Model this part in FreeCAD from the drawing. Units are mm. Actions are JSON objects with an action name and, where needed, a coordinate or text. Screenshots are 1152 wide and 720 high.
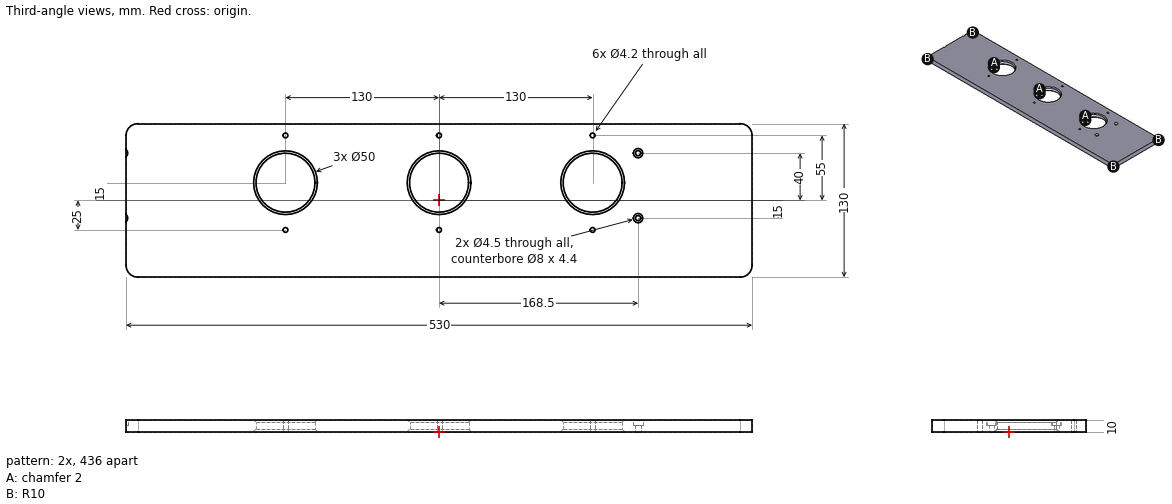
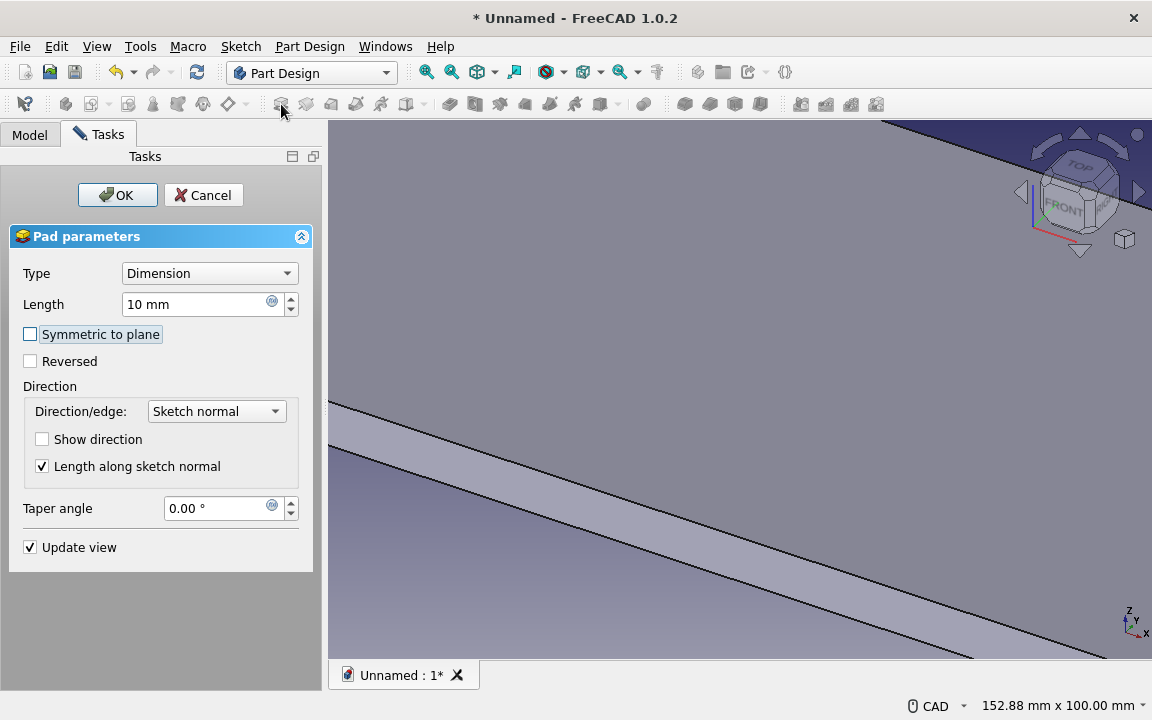
{"action": "left_click", "coordinate": [118, 195]}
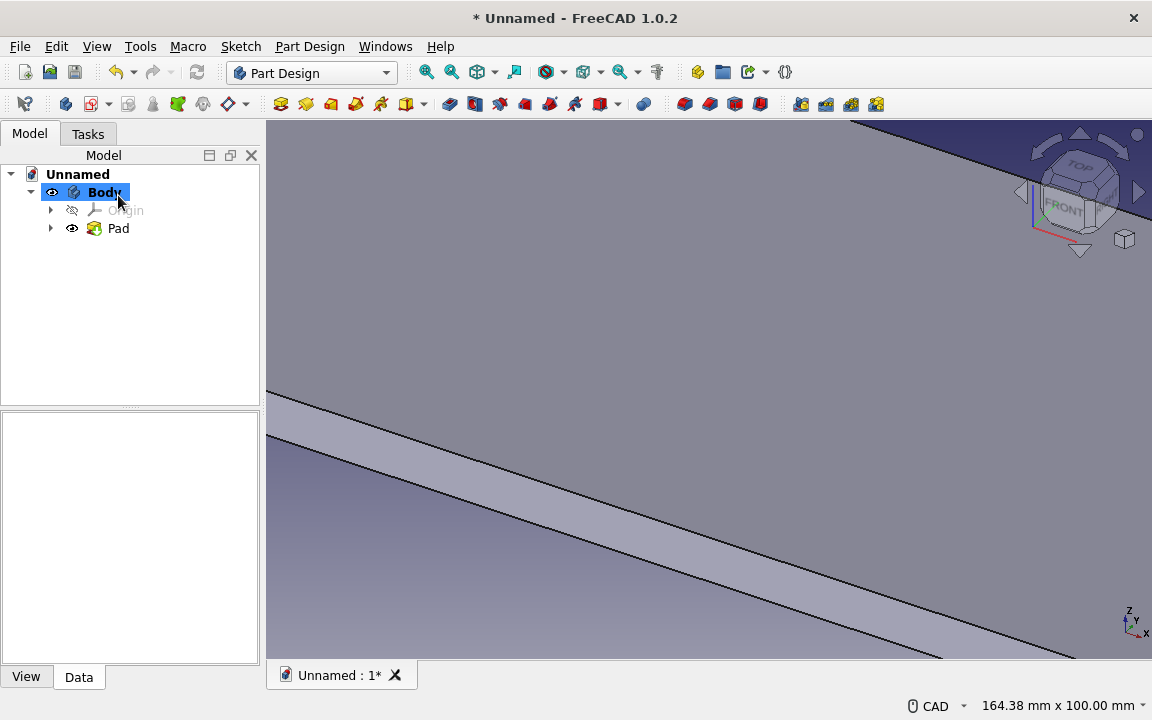
{"action": "left_click", "coordinate": [427, 72]}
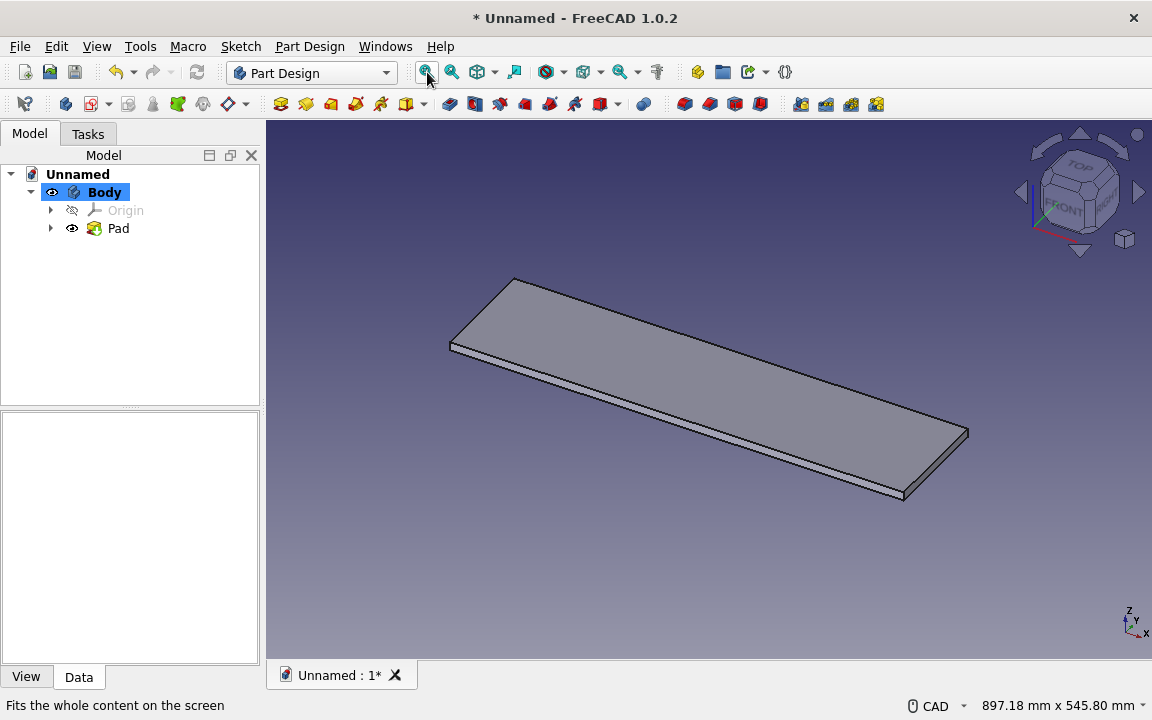
{"action": "left_click", "coordinate": [839, 427]}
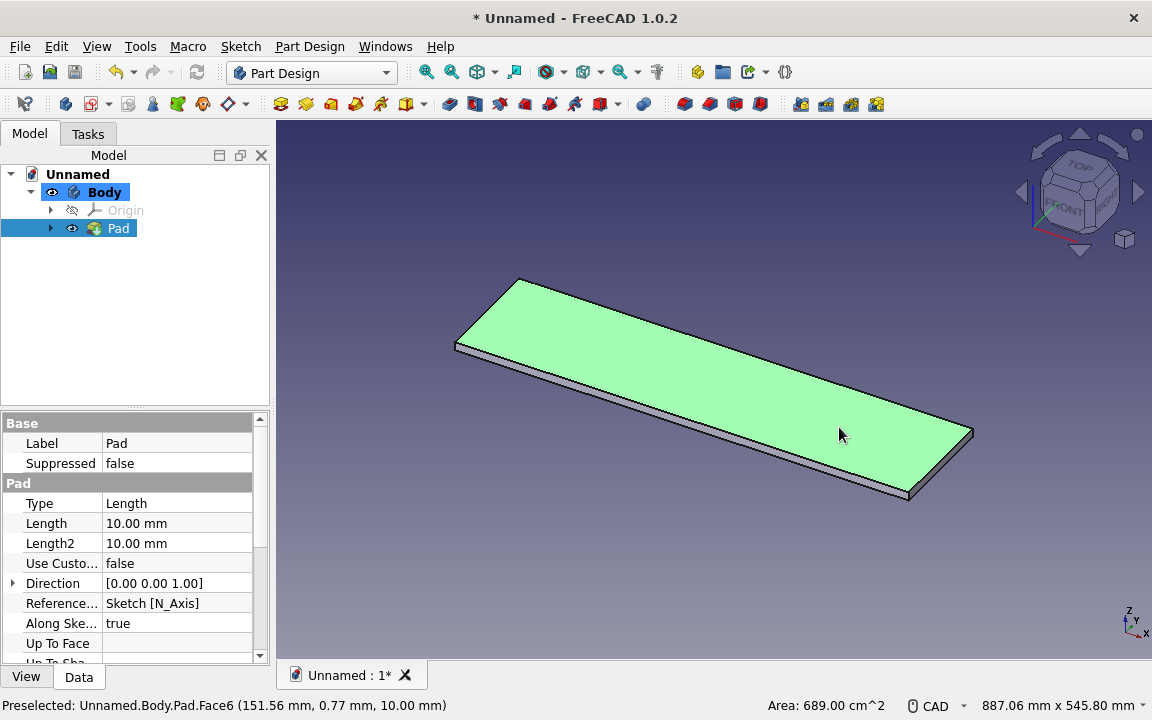
{"action": "left_click", "coordinate": [90, 104]}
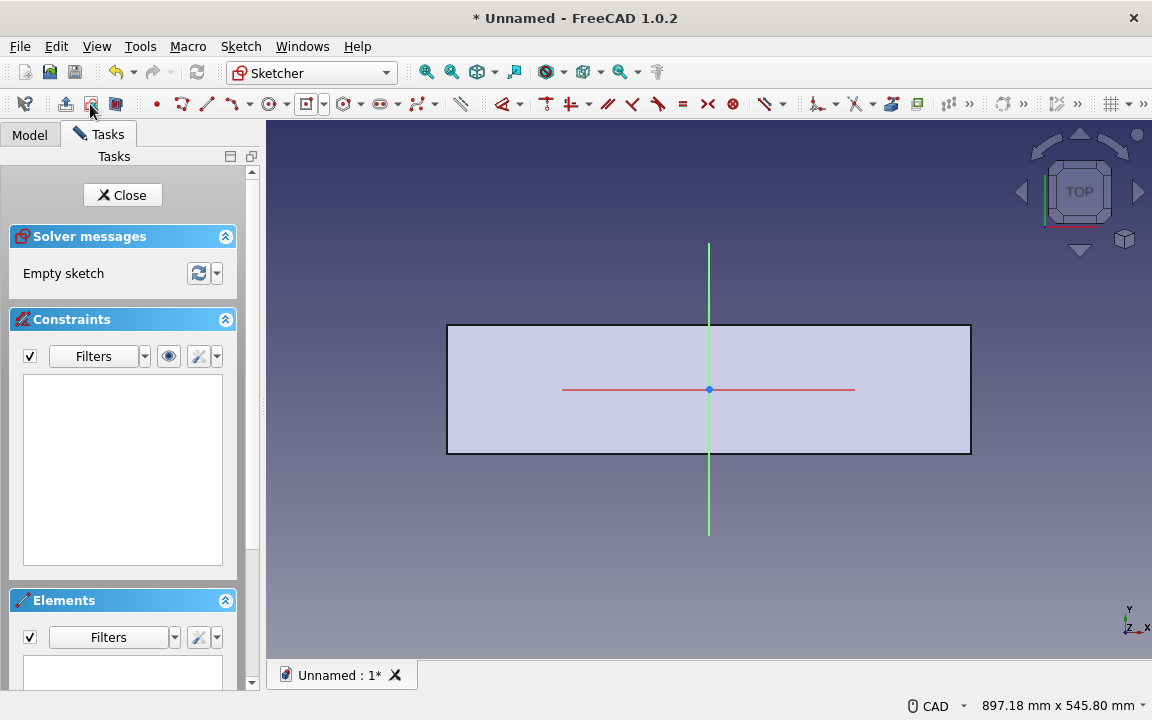
{"action": "scroll", "coordinate": [922, 375], "scroll_direction": "up", "scroll_amount": 9}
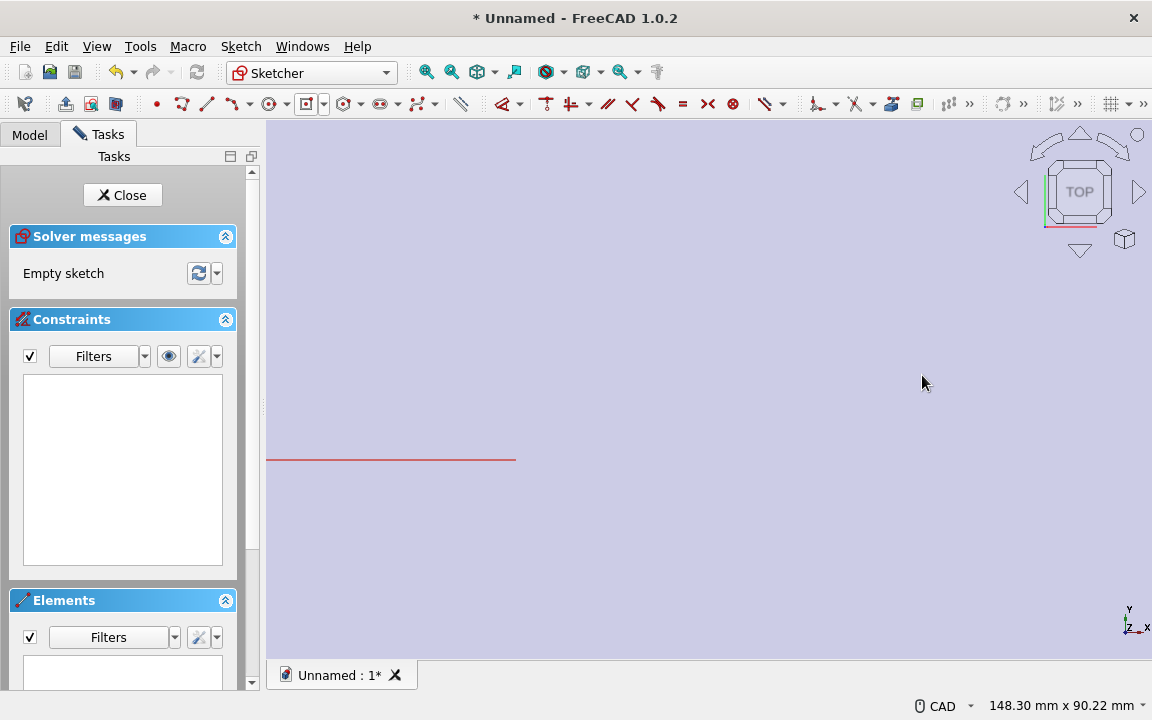
{"action": "left_click", "coordinate": [268, 104]}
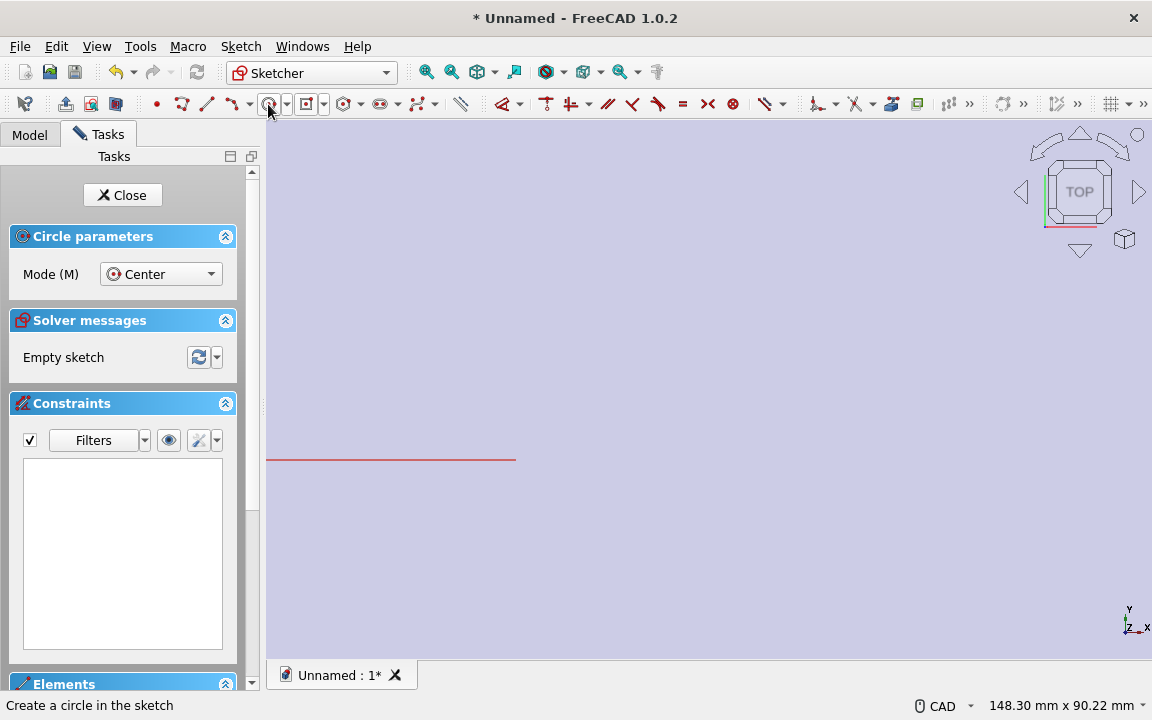
{"action": "scroll", "coordinate": [636, 550], "scroll_direction": "up", "scroll_amount": 3}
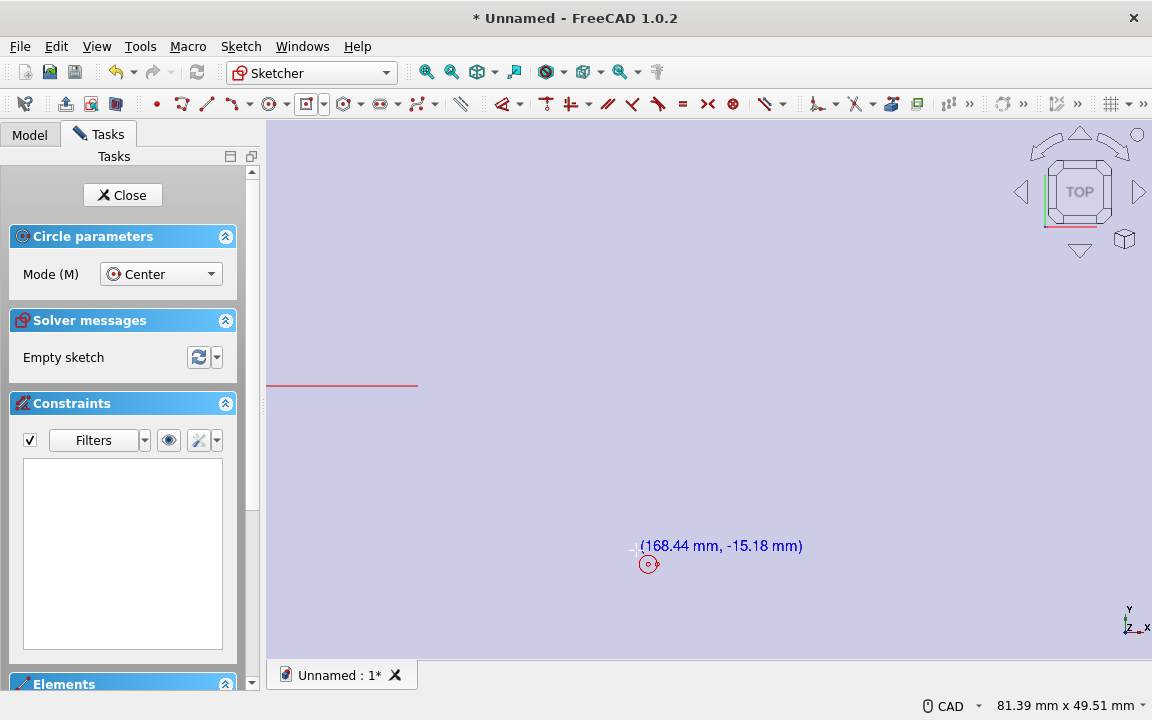
{"action": "left_click", "coordinate": [636, 549]}
{"action": "mouse_move", "coordinate": [654, 532]}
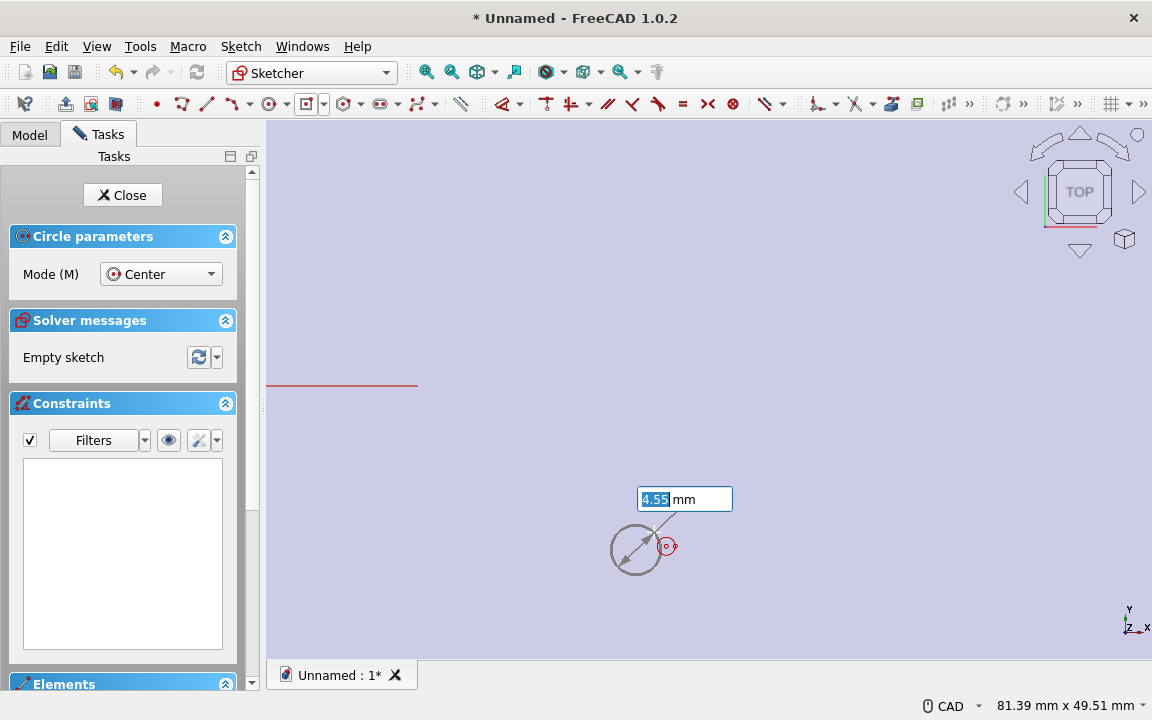
{"action": "type", "text": "4.5"}
{"action": "key", "text": "Return"}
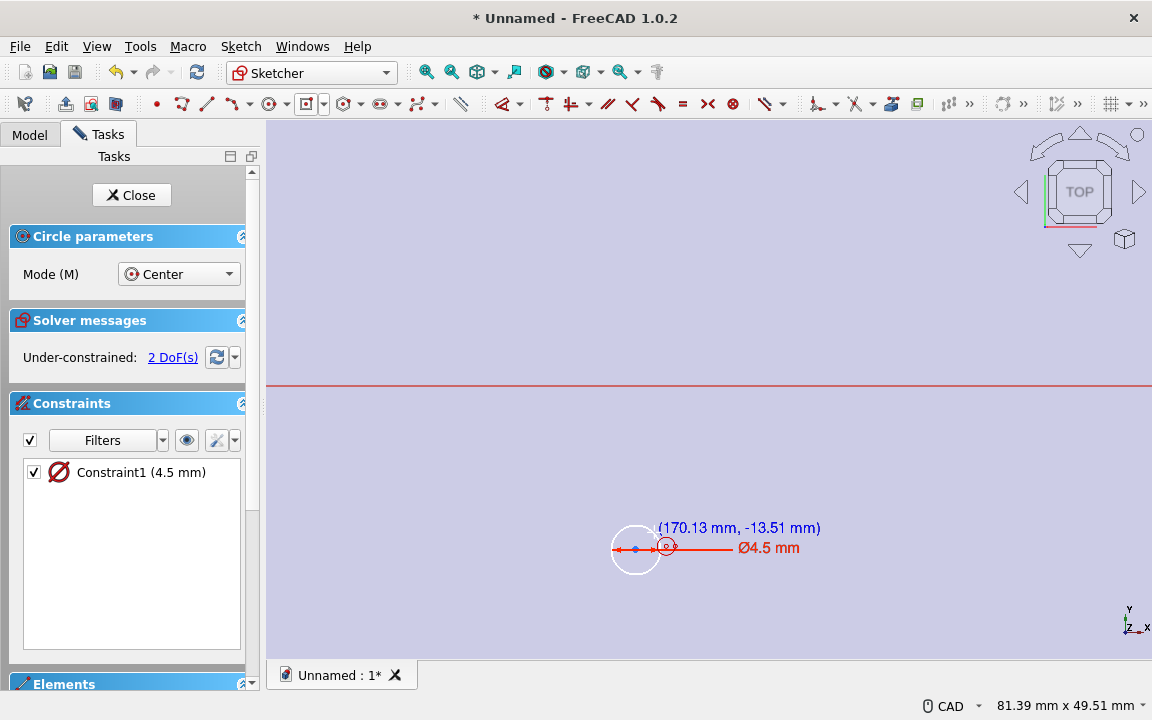
{"action": "scroll", "coordinate": [646, 559], "scroll_direction": "down", "scroll_amount": 3}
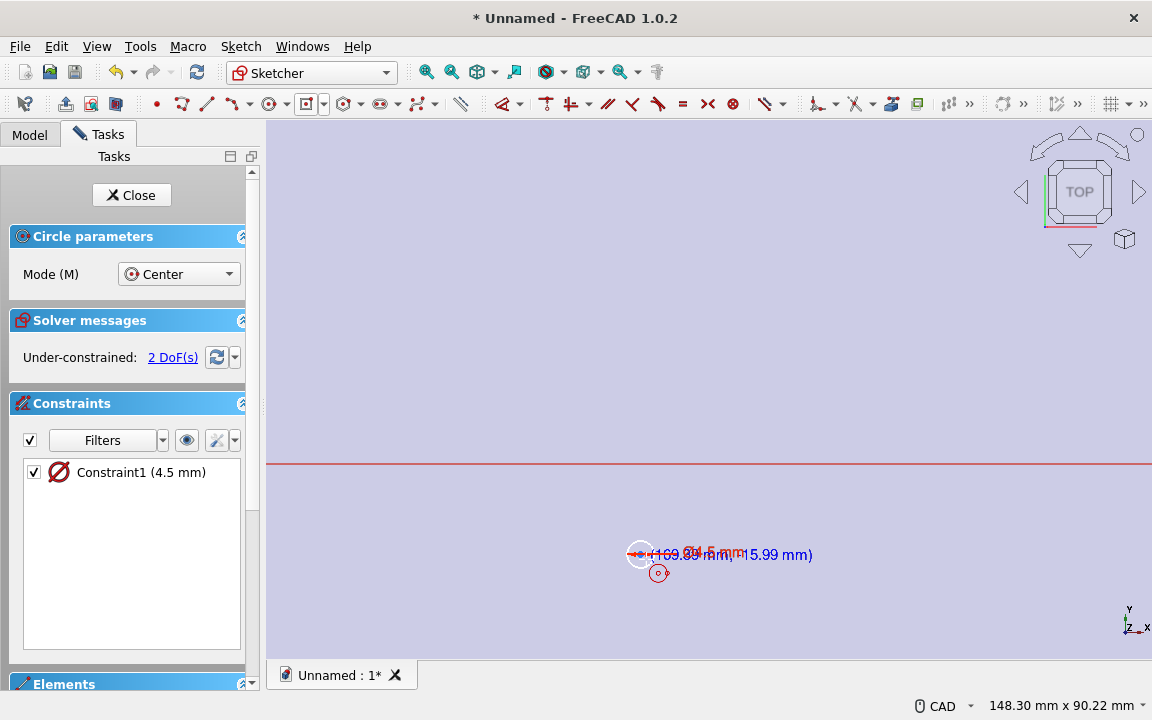
{"action": "scroll", "coordinate": [641, 225], "scroll_direction": "up", "scroll_amount": 3}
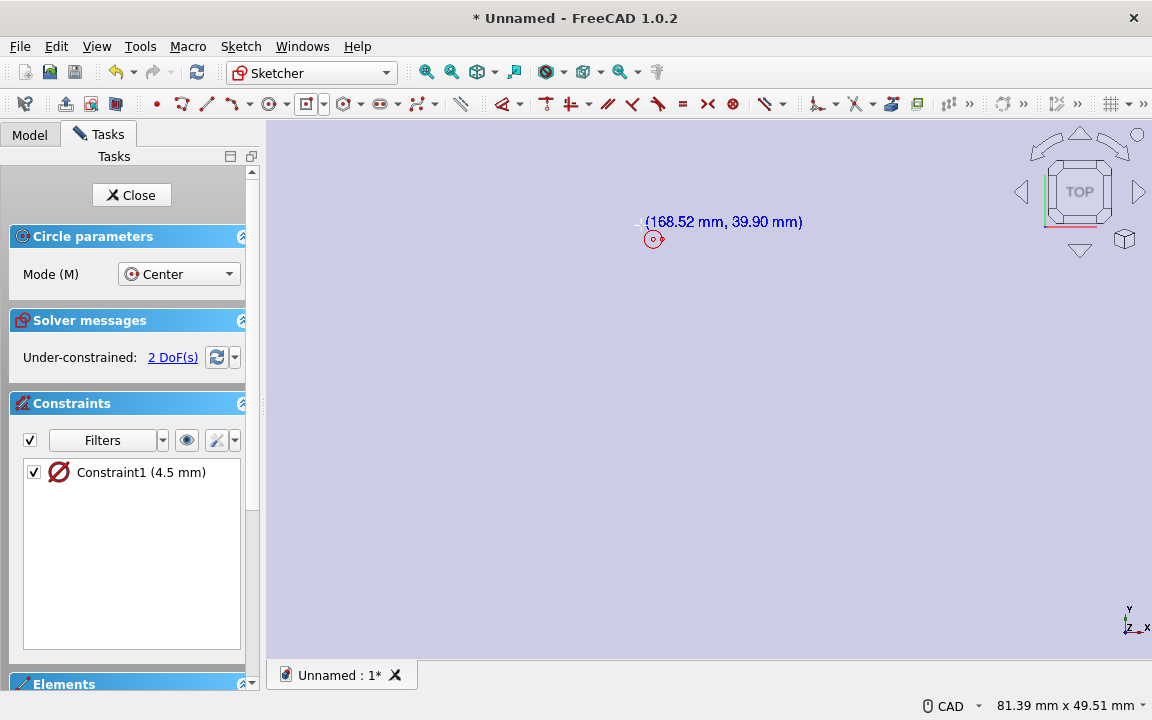
{"action": "left_click", "coordinate": [640, 226]}
{"action": "mouse_move", "coordinate": [658, 208]}